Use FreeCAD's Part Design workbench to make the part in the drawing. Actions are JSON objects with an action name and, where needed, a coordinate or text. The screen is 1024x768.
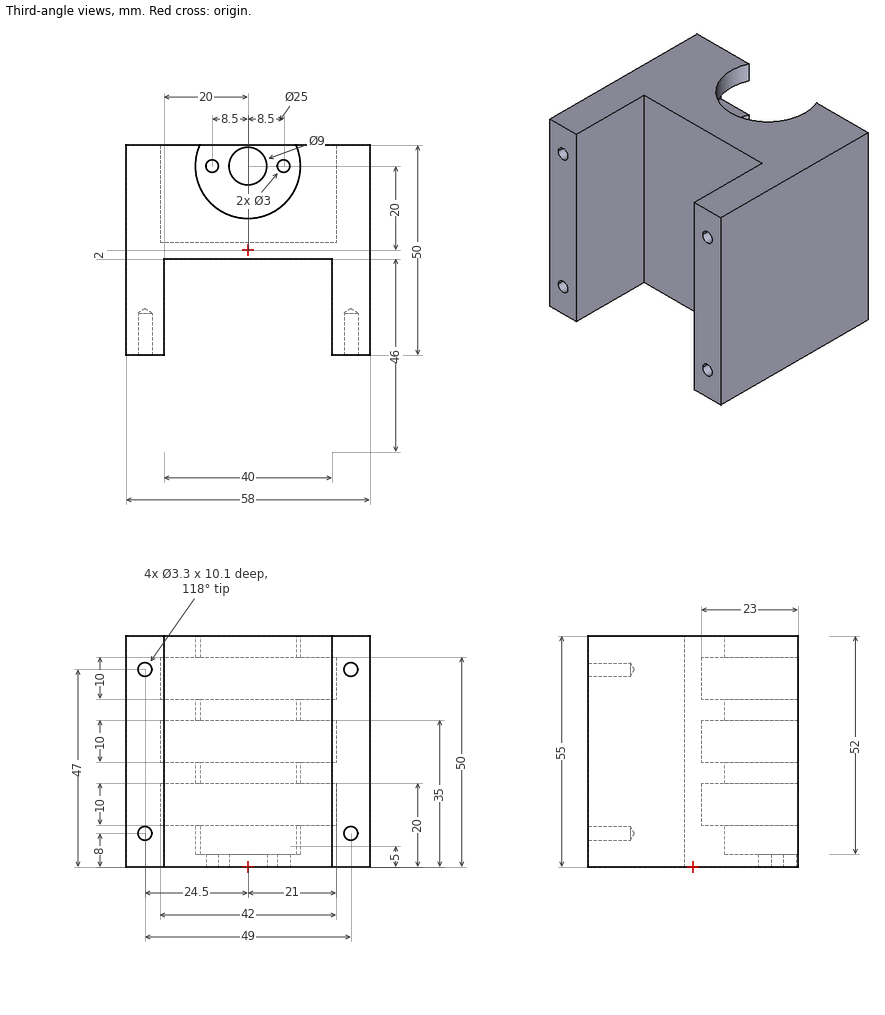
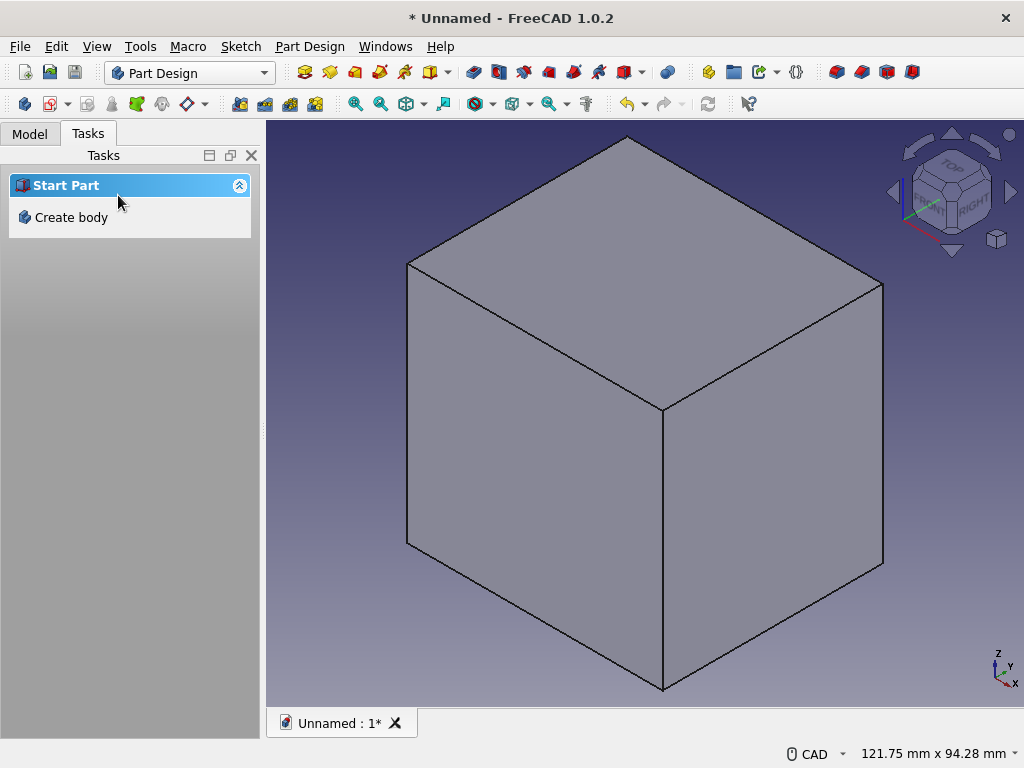
{"action": "left_click", "coordinate": [645, 273]}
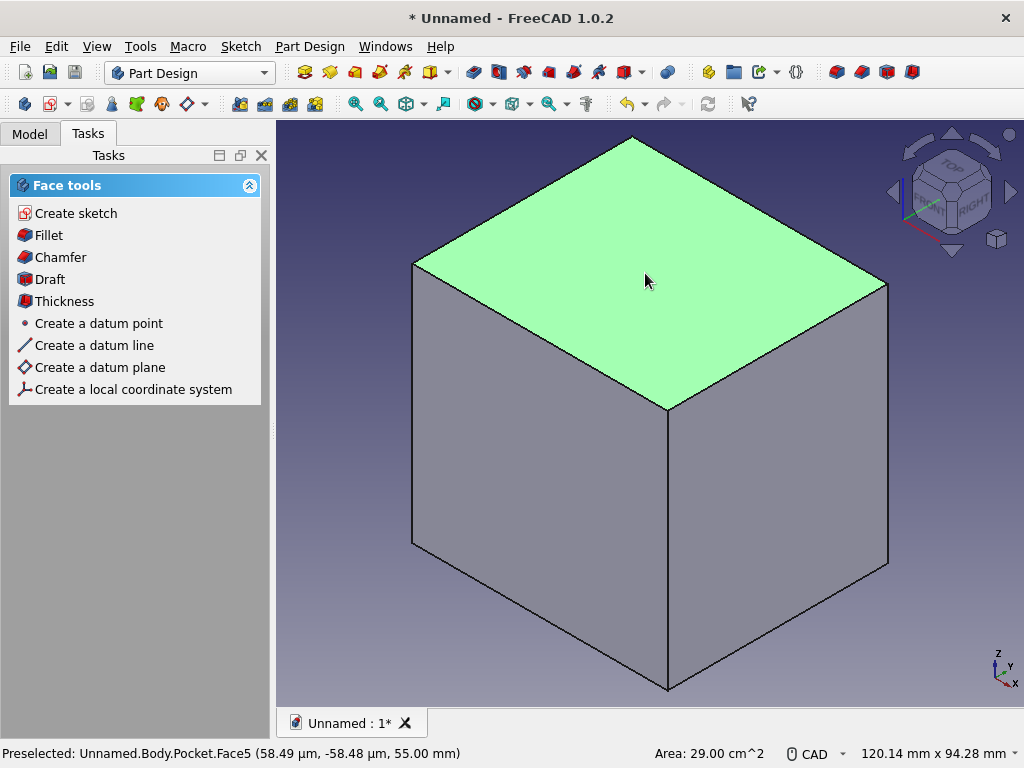
{"action": "left_click", "coordinate": [50, 104]}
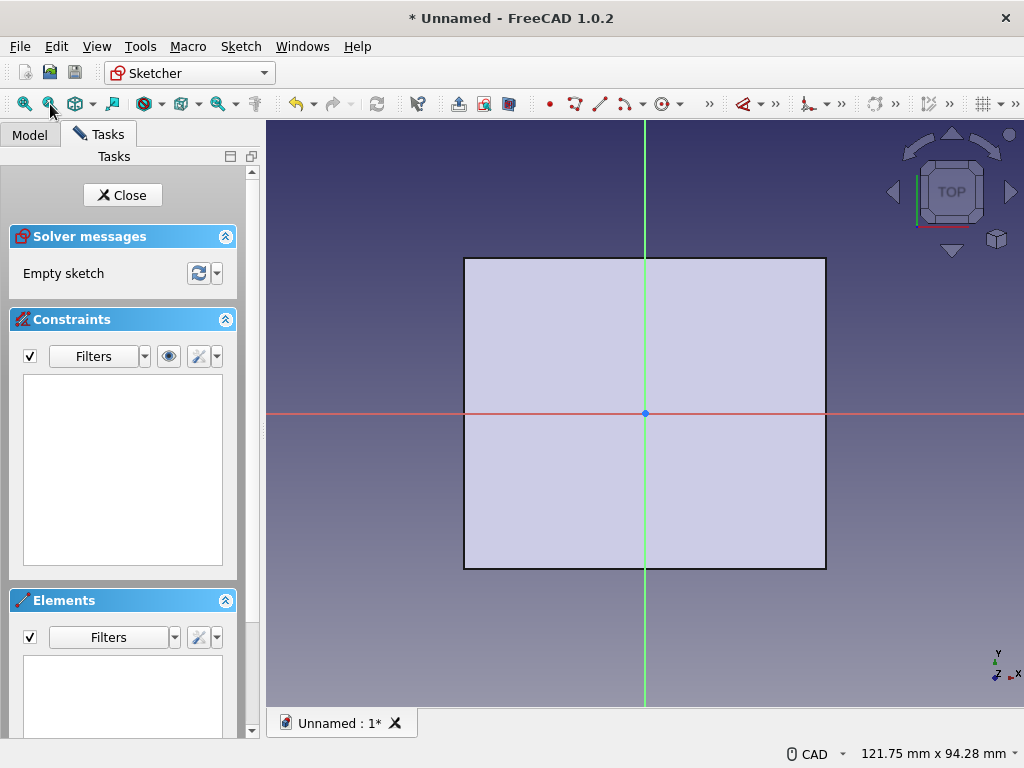
{"action": "scroll", "coordinate": [728, 189], "scroll_direction": "up", "scroll_amount": 3}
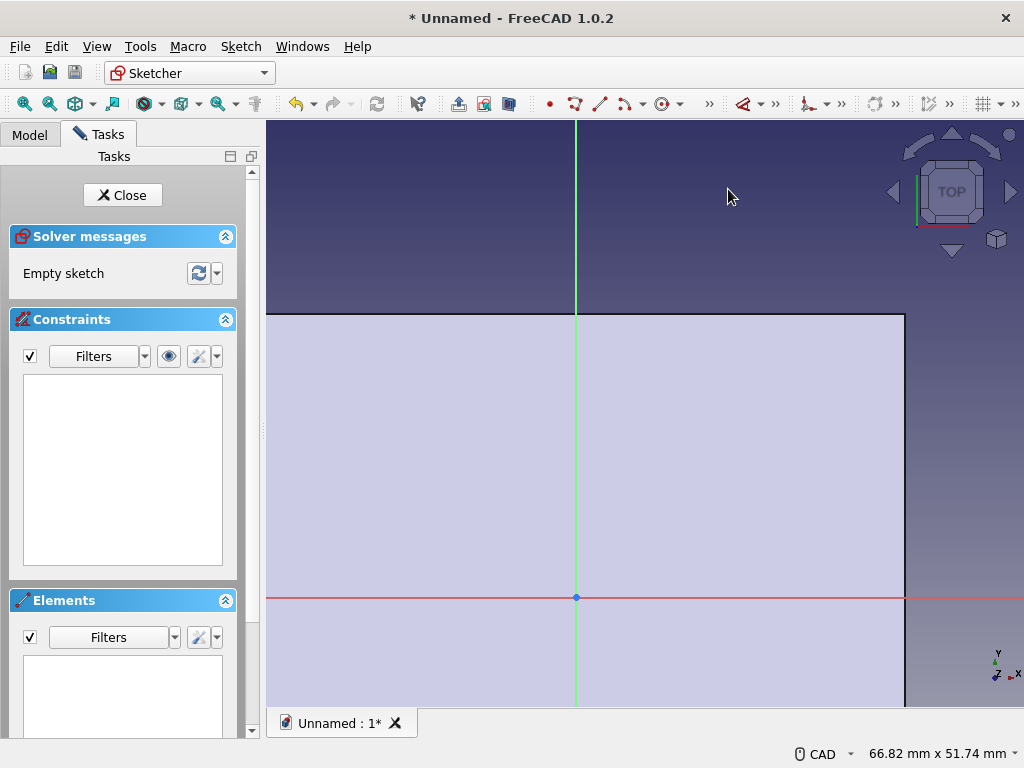
{"action": "left_click", "coordinate": [662, 104]}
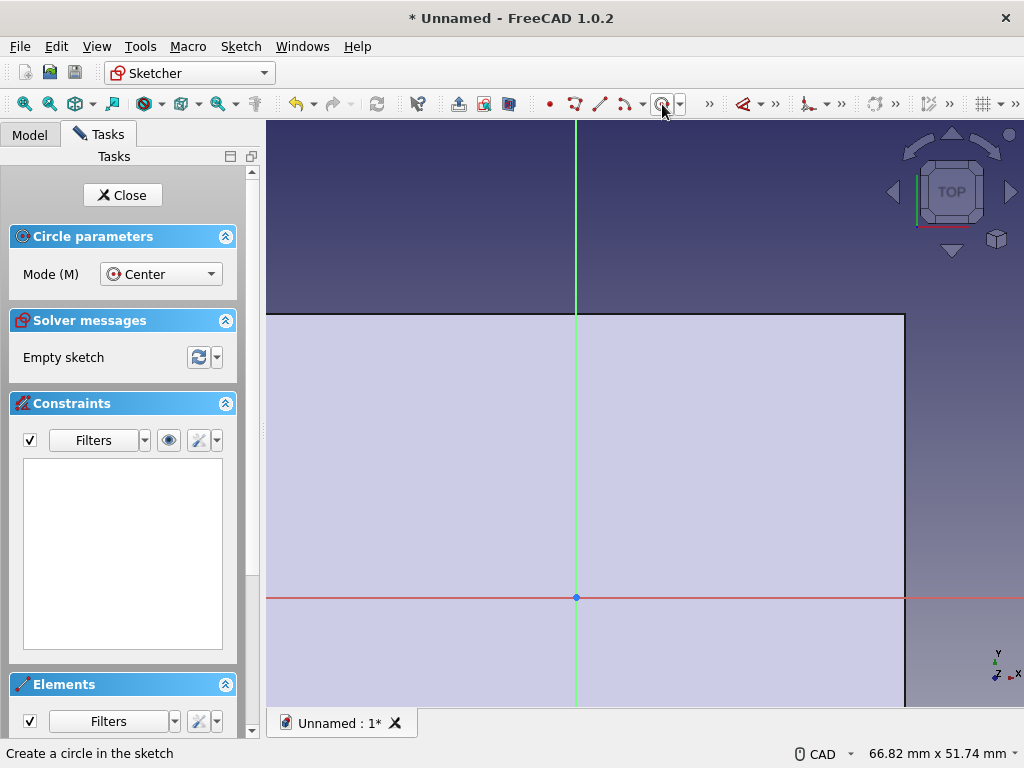
{"action": "left_click", "coordinate": [576, 371]}
{"action": "mouse_move", "coordinate": [677, 271]}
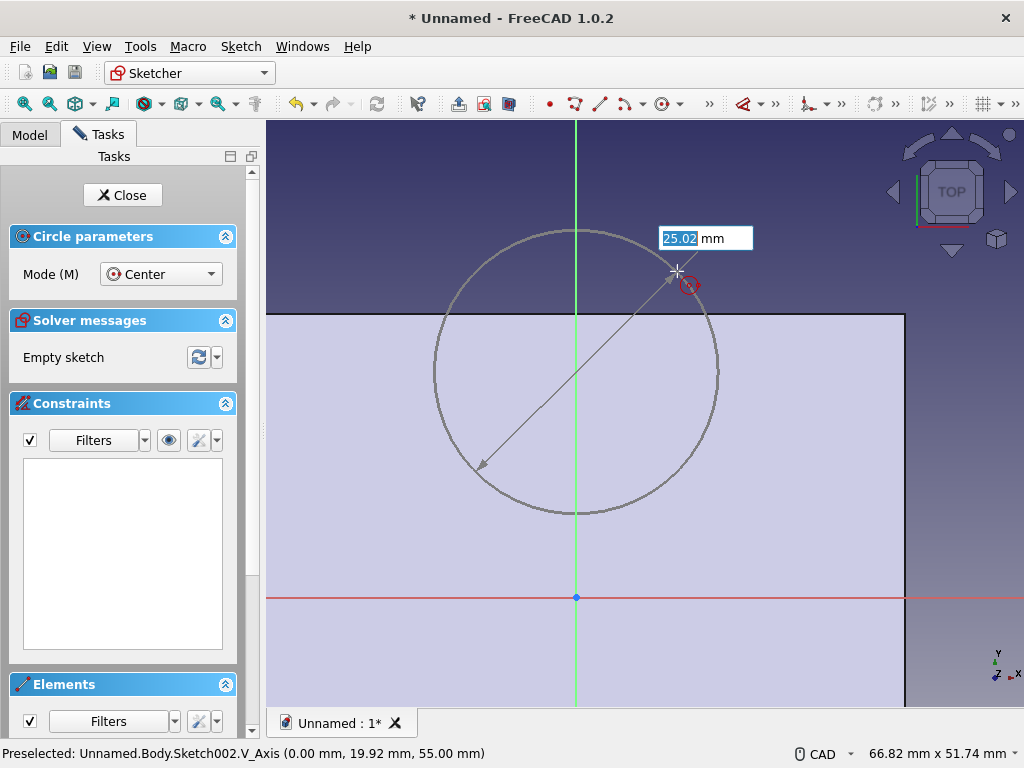
{"action": "type", "text": "25"}
{"action": "key", "text": "Return"}
{"action": "key", "text": "Escape"}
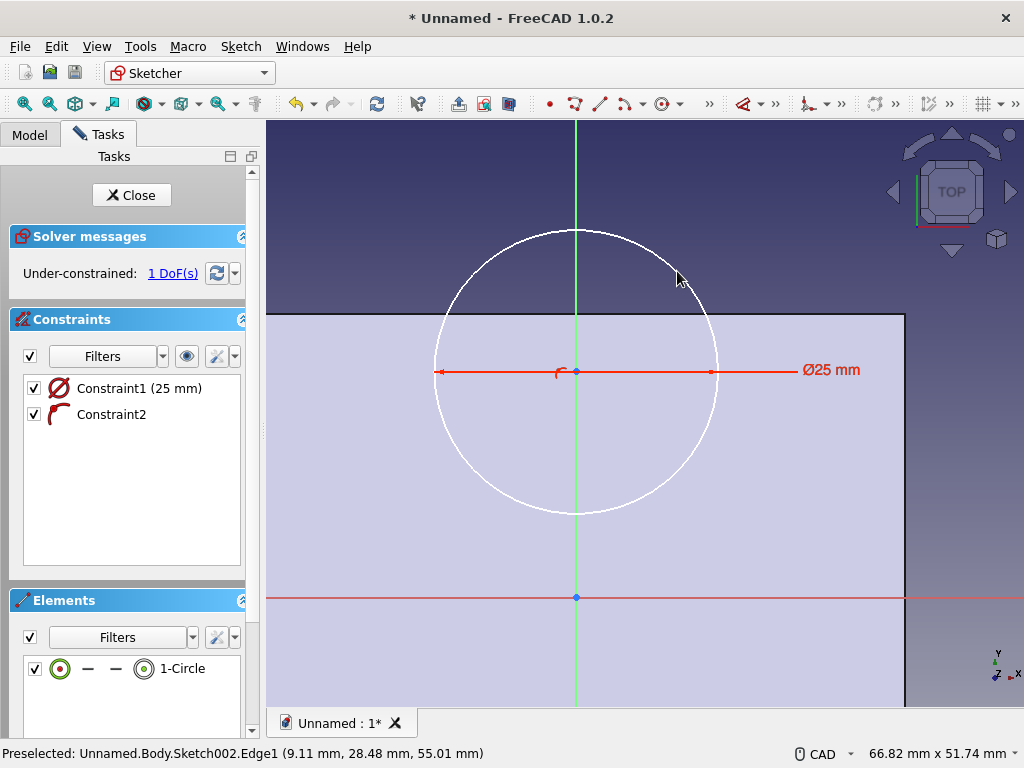
{"action": "left_click", "coordinate": [742, 104]}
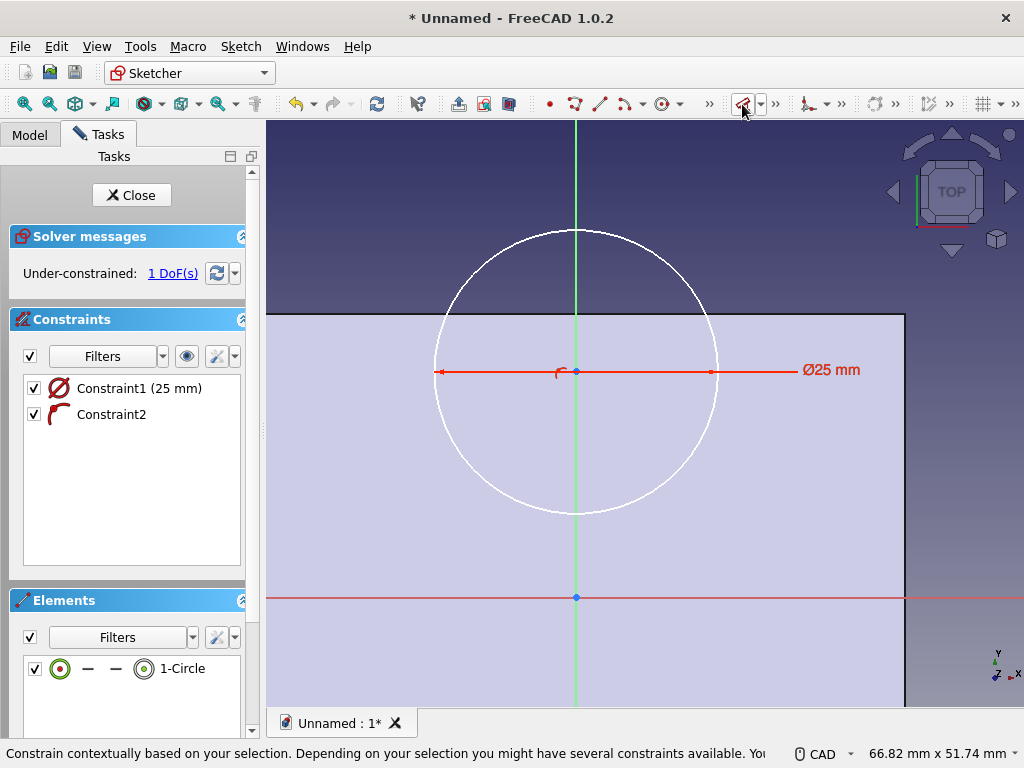
{"action": "left_click", "coordinate": [576, 372]}
{"action": "left_click", "coordinate": [610, 485]}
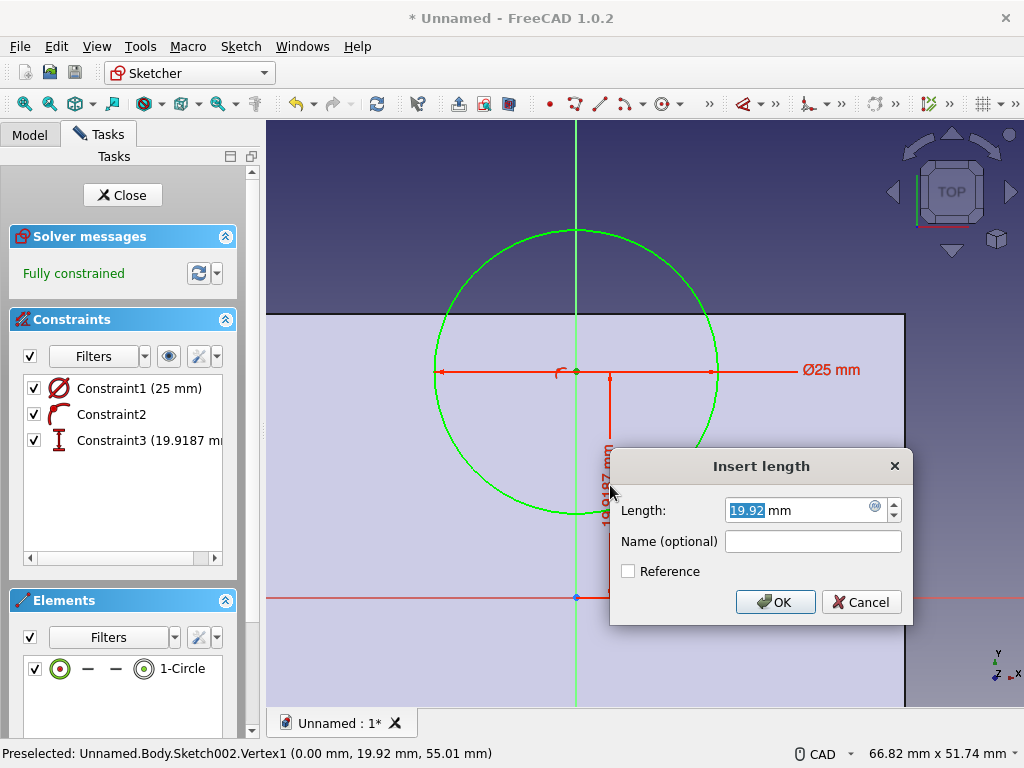
{"action": "type", "text": "20"}
{"action": "key", "text": "Return"}
{"action": "key", "text": "Escape"}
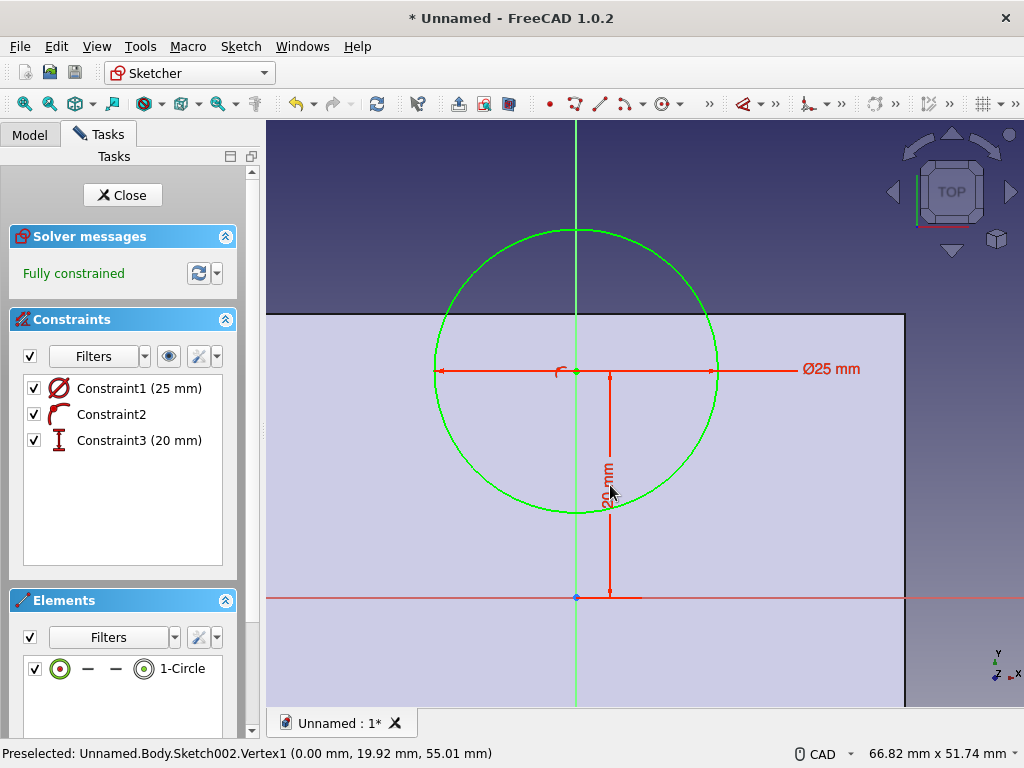
{"action": "left_click", "coordinate": [123, 195]}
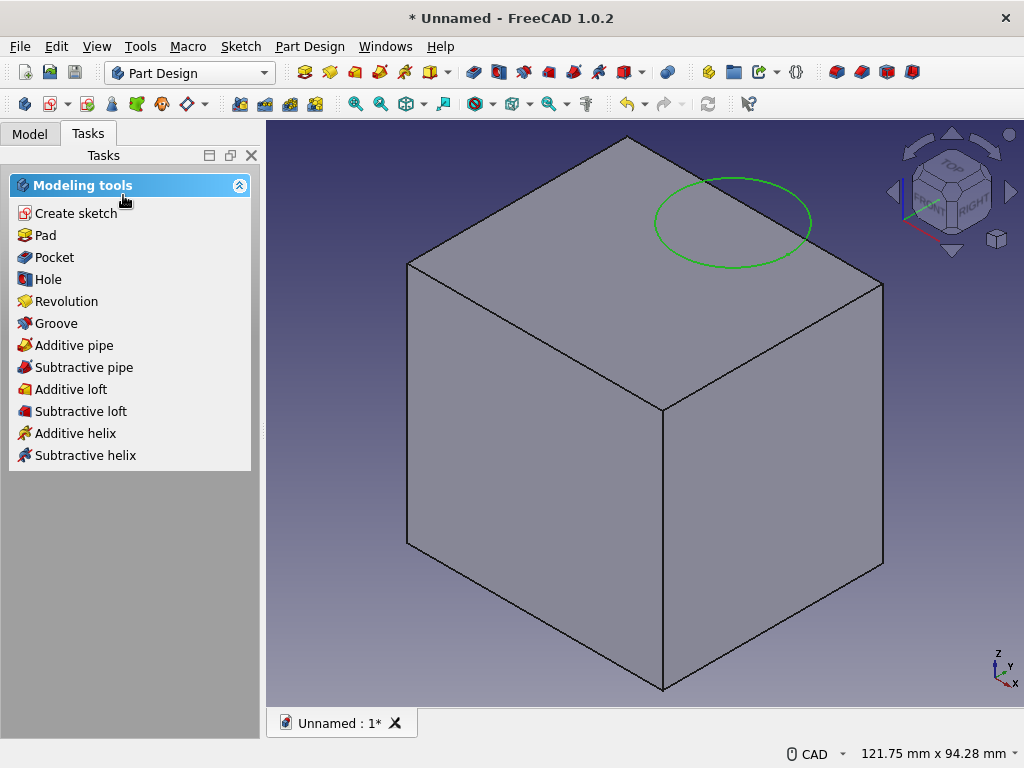
{"action": "left_click", "coordinate": [474, 72]}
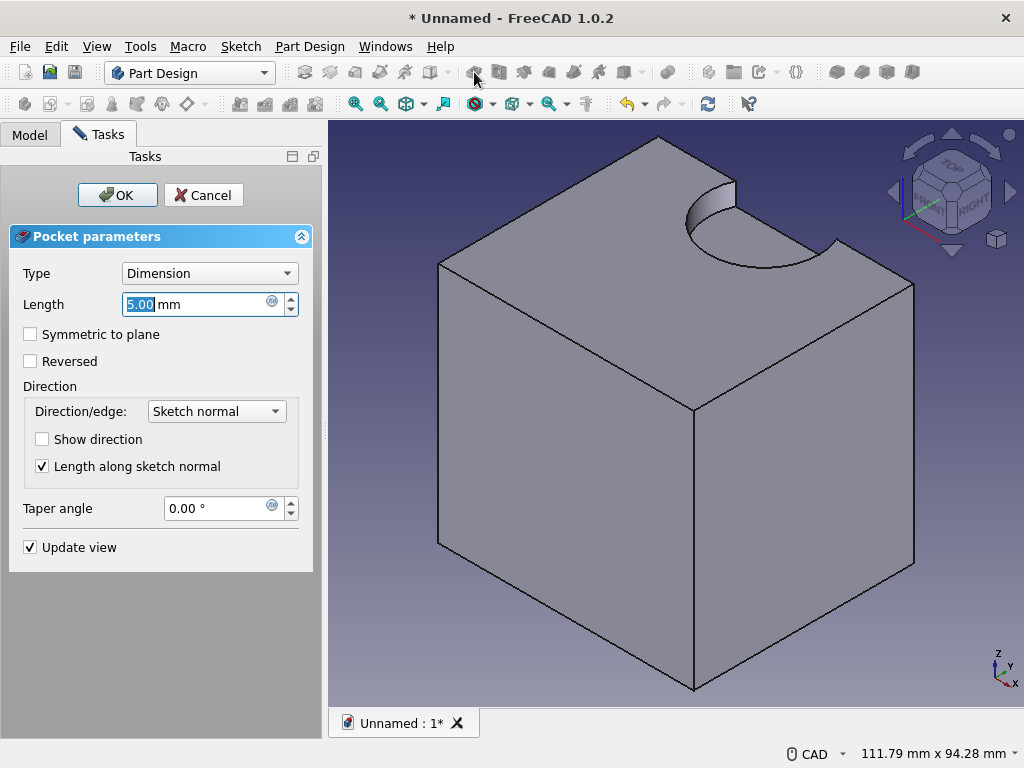
{"action": "type", "text": "52"}
{"action": "key", "text": "Tab"}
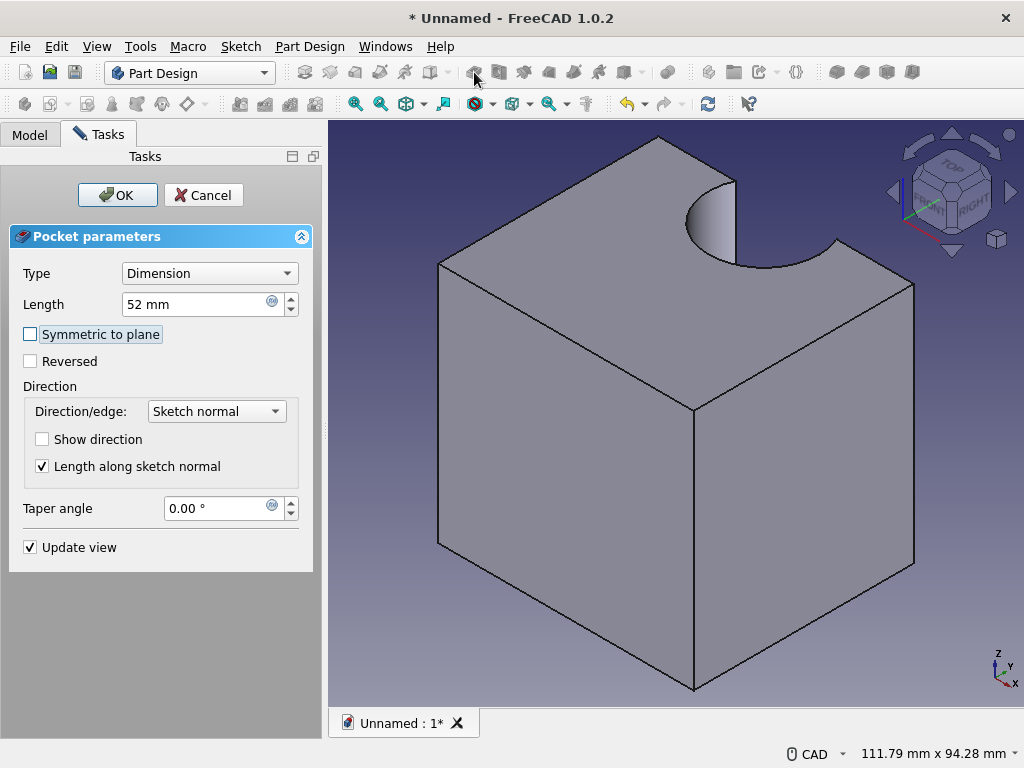
{"action": "left_click", "coordinate": [118, 195]}